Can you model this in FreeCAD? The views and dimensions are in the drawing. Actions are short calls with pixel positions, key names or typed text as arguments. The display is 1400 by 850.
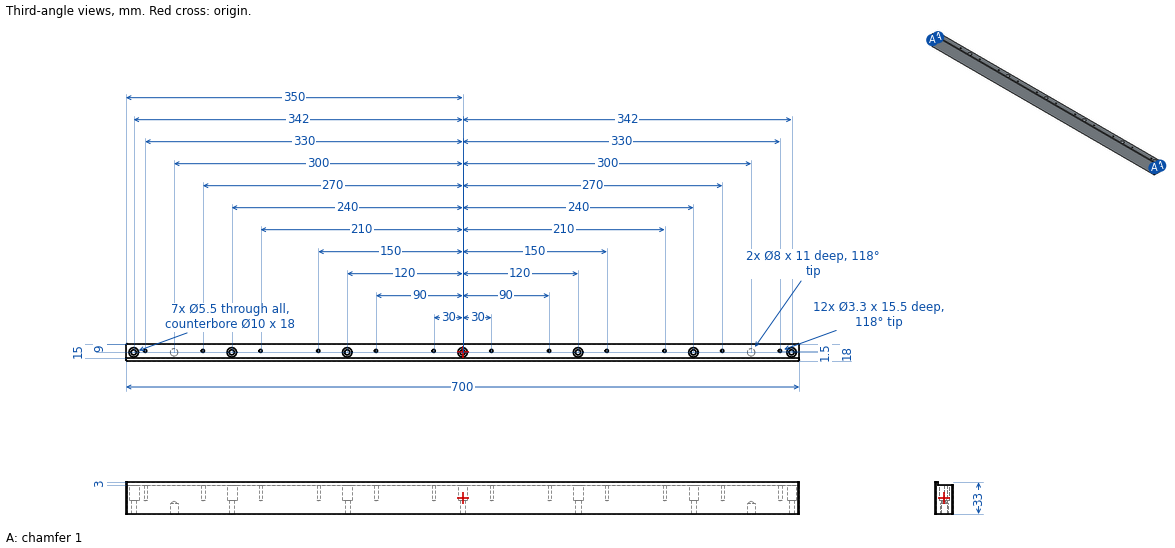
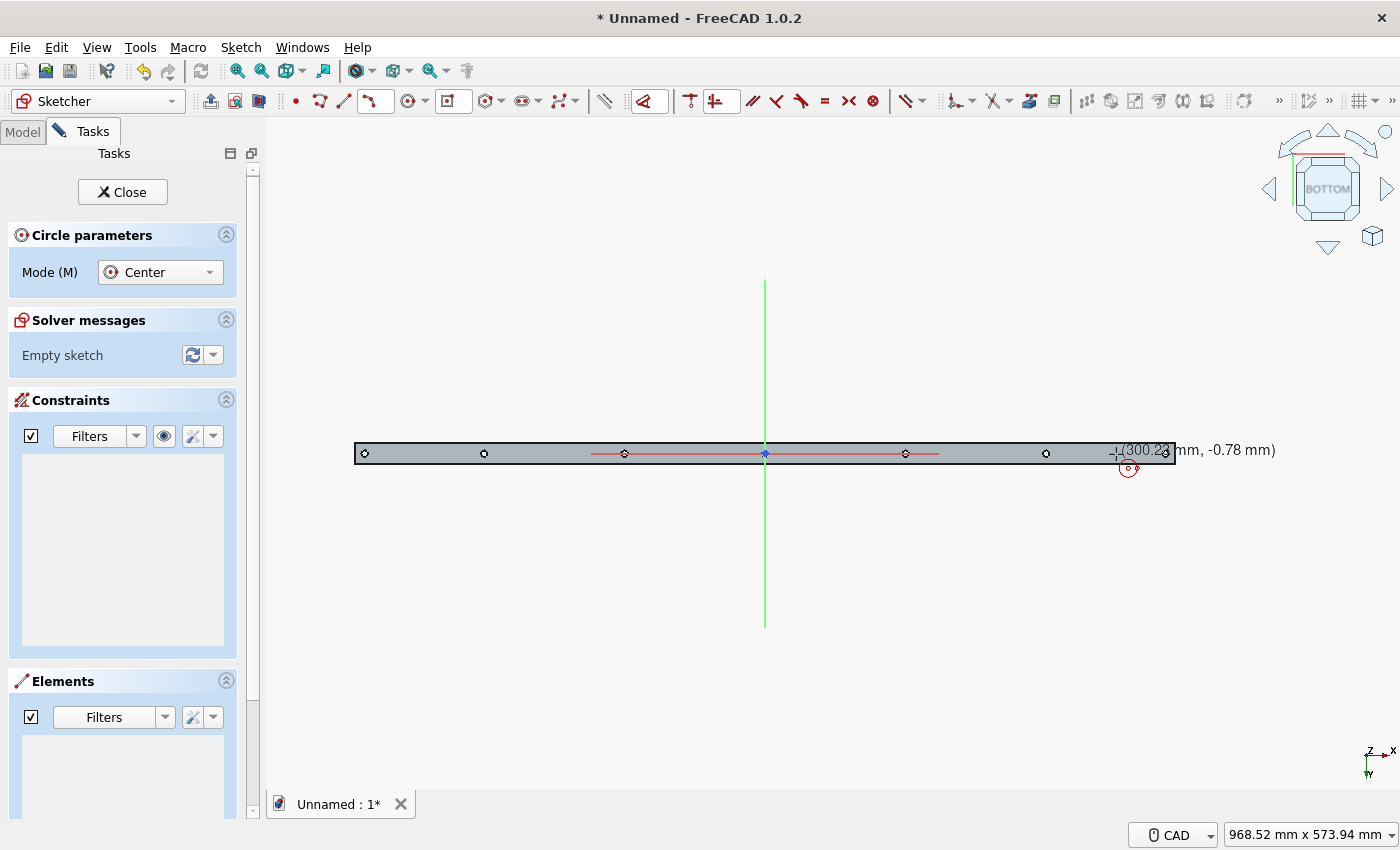
click(1116, 454)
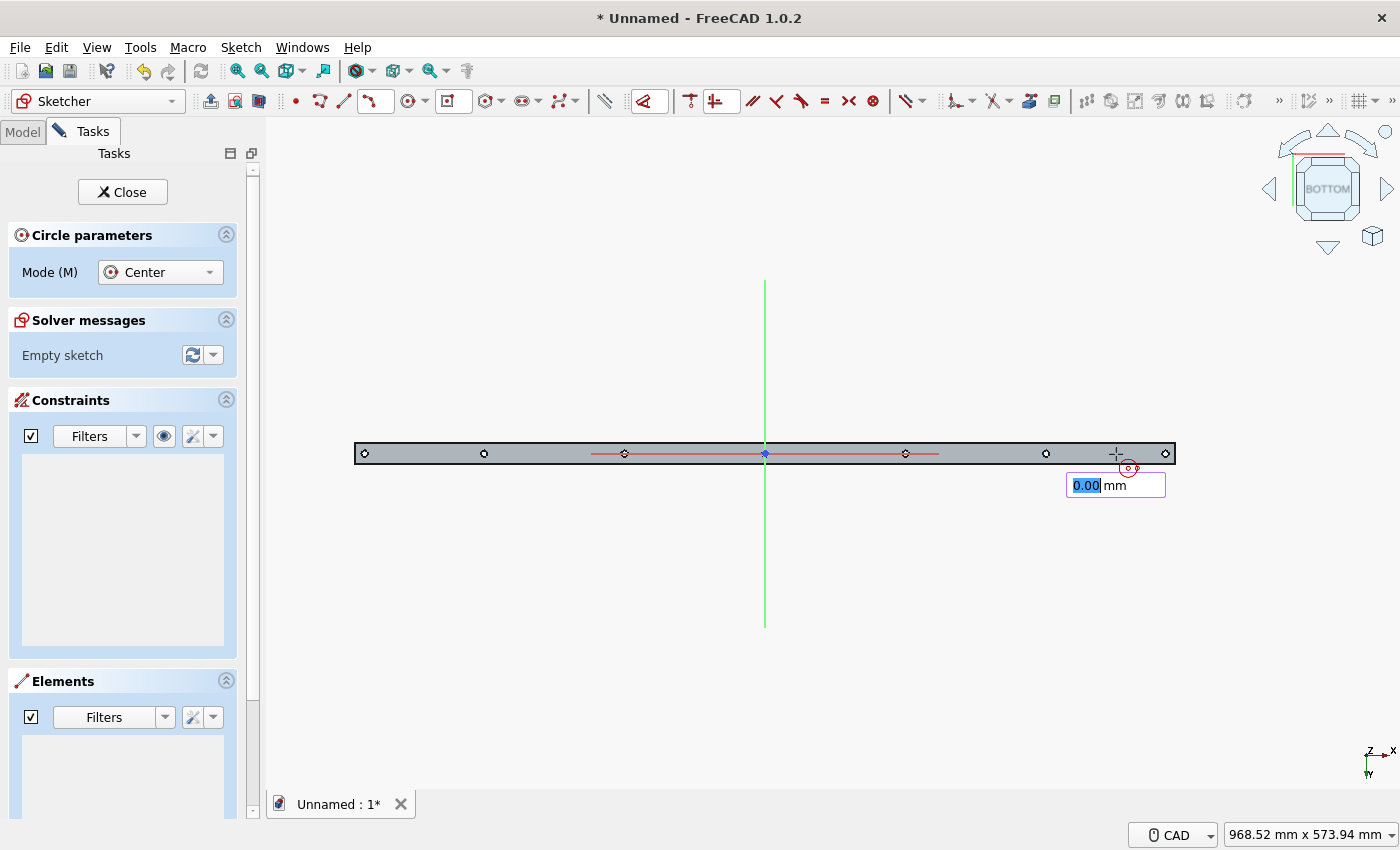
scroll(1115, 458, up, 7)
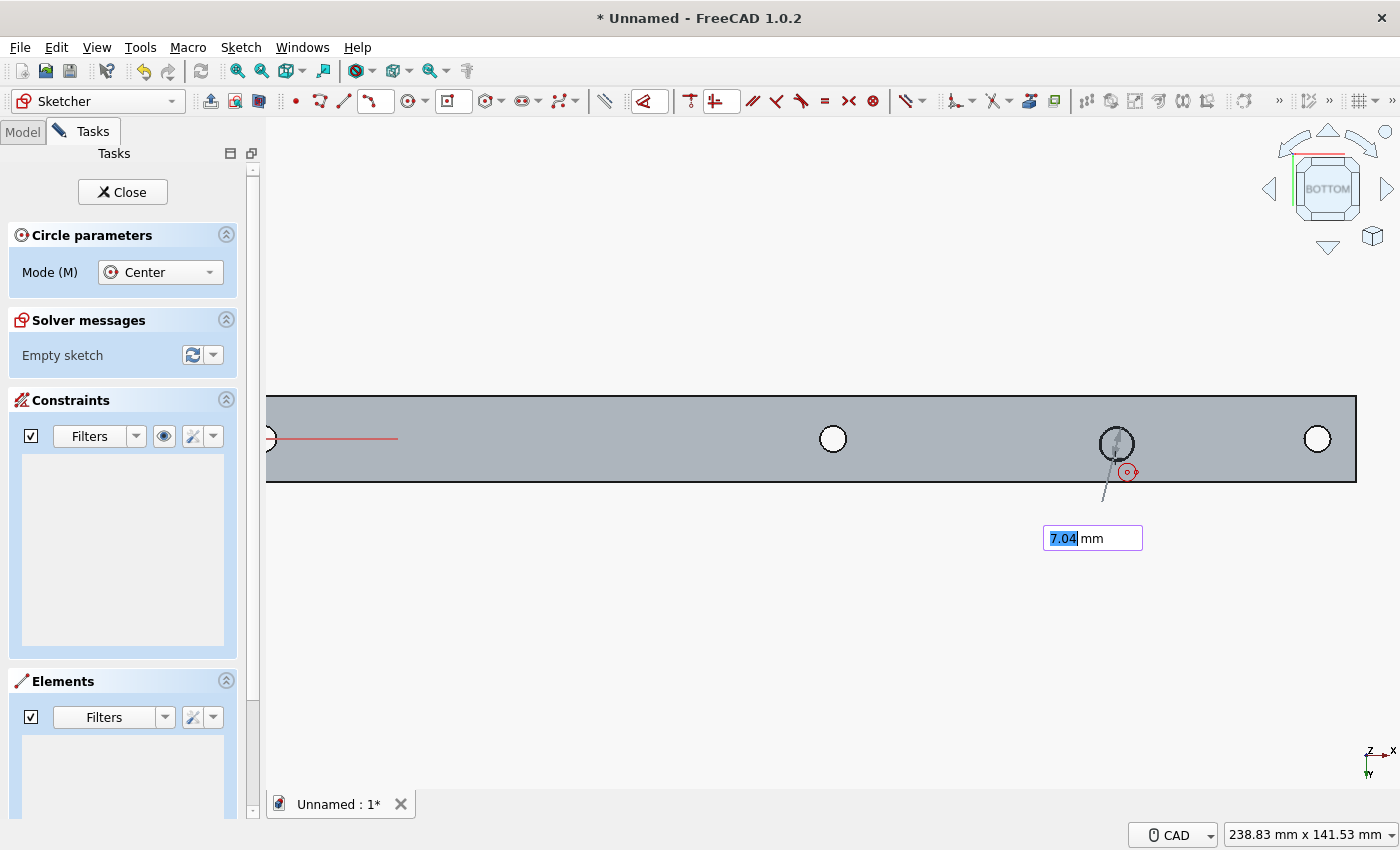
click(1112, 457)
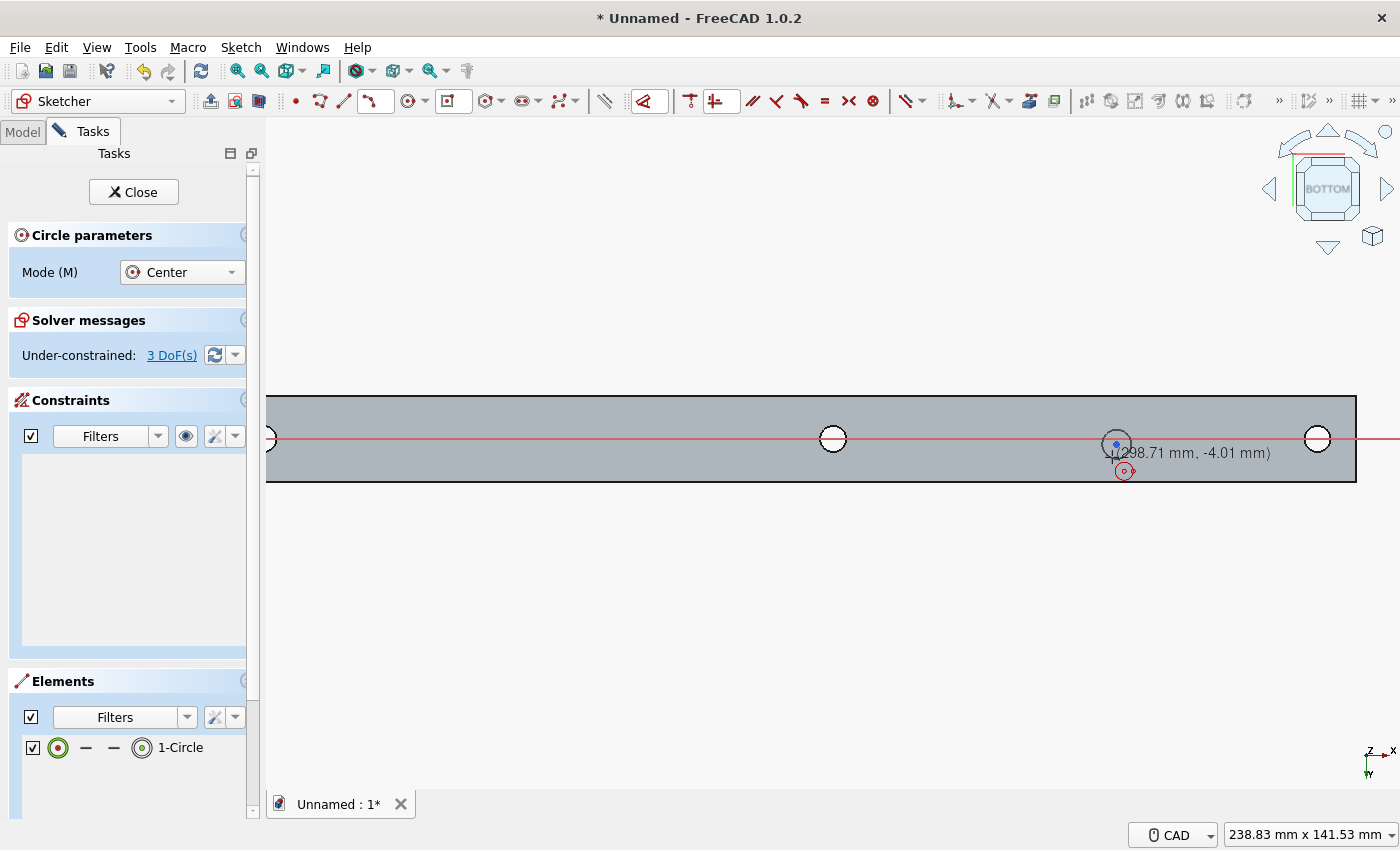
scroll(1115, 458, down, 7)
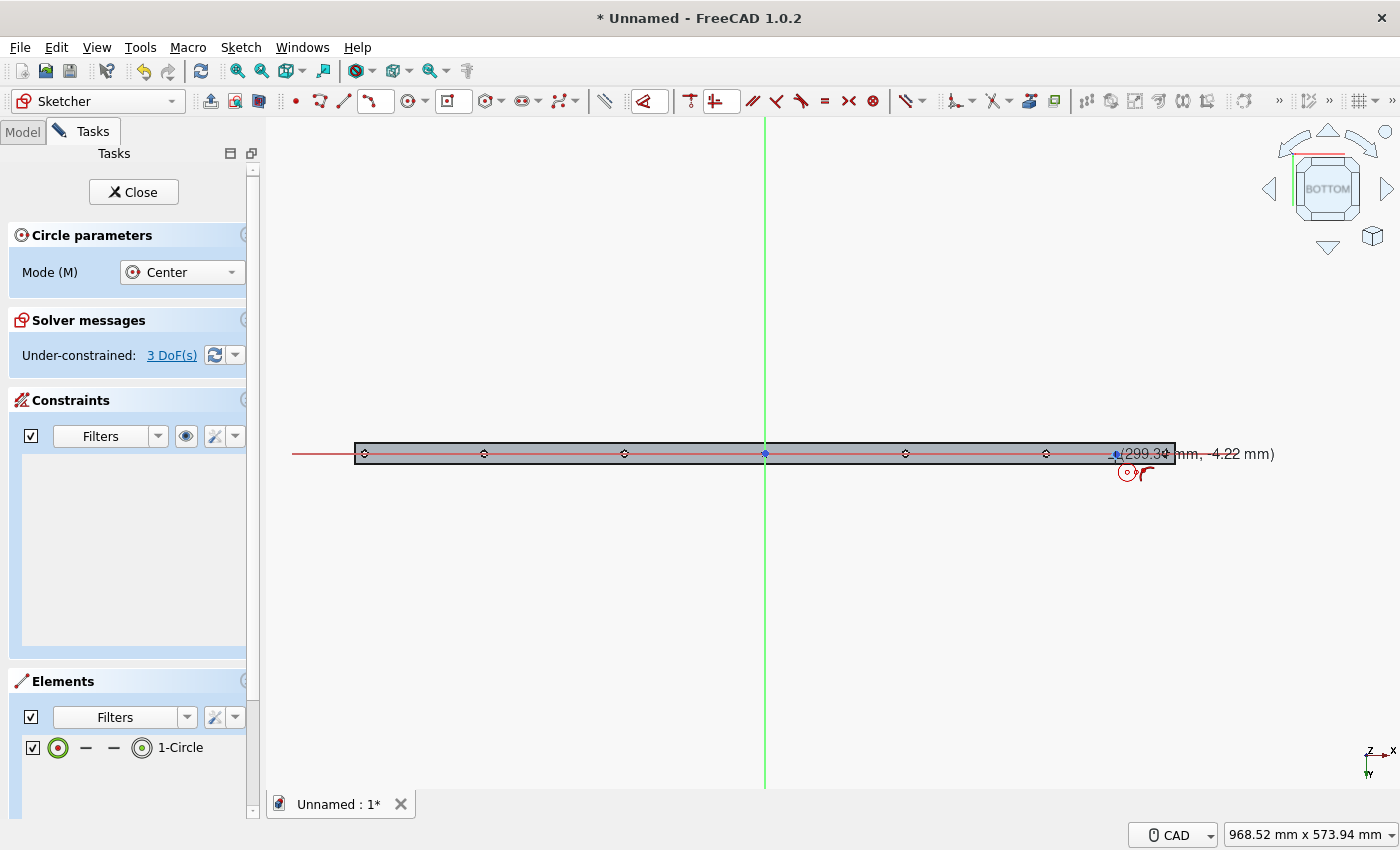
scroll(414, 454, up, 8)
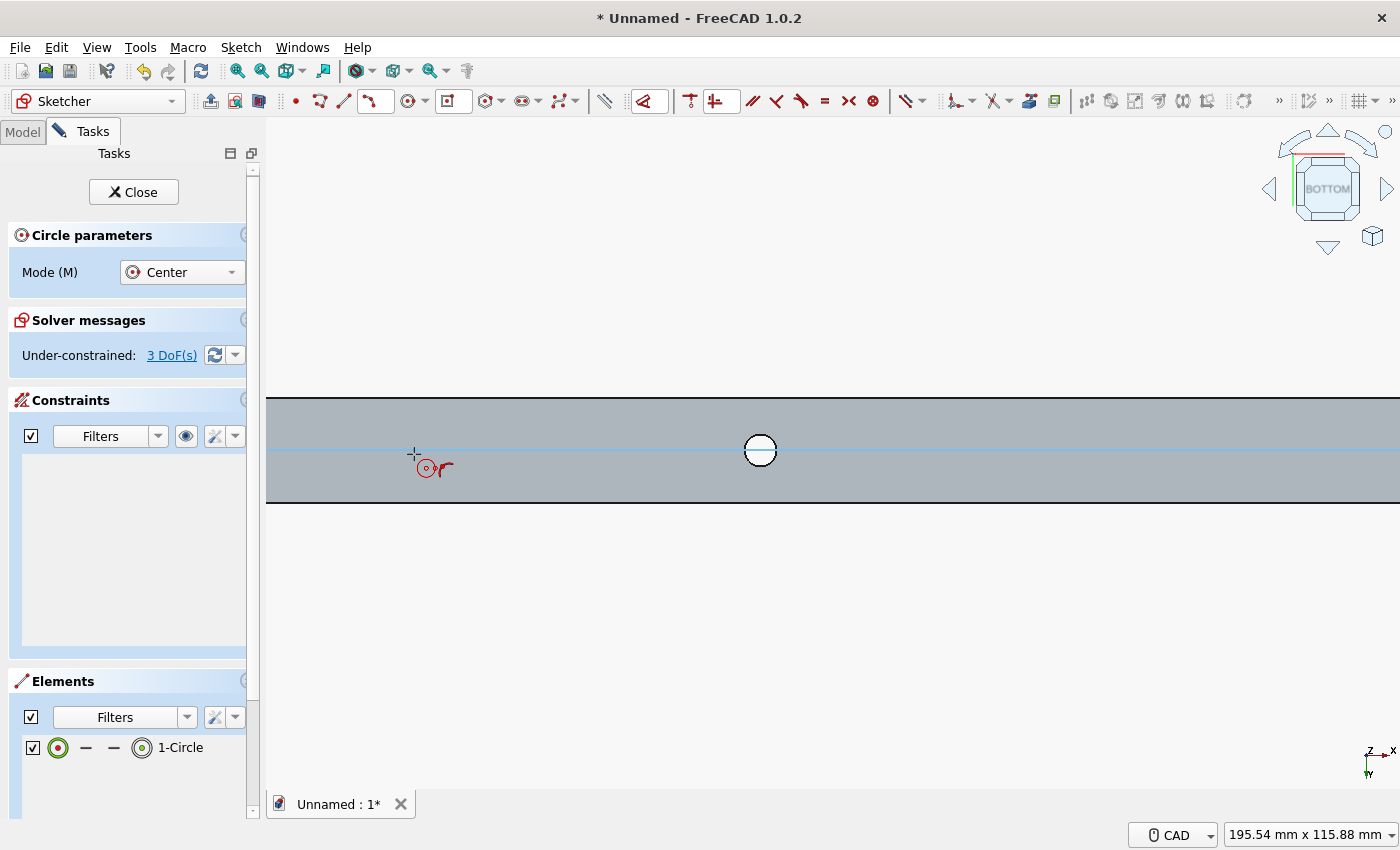
scroll(413, 454, down, 8)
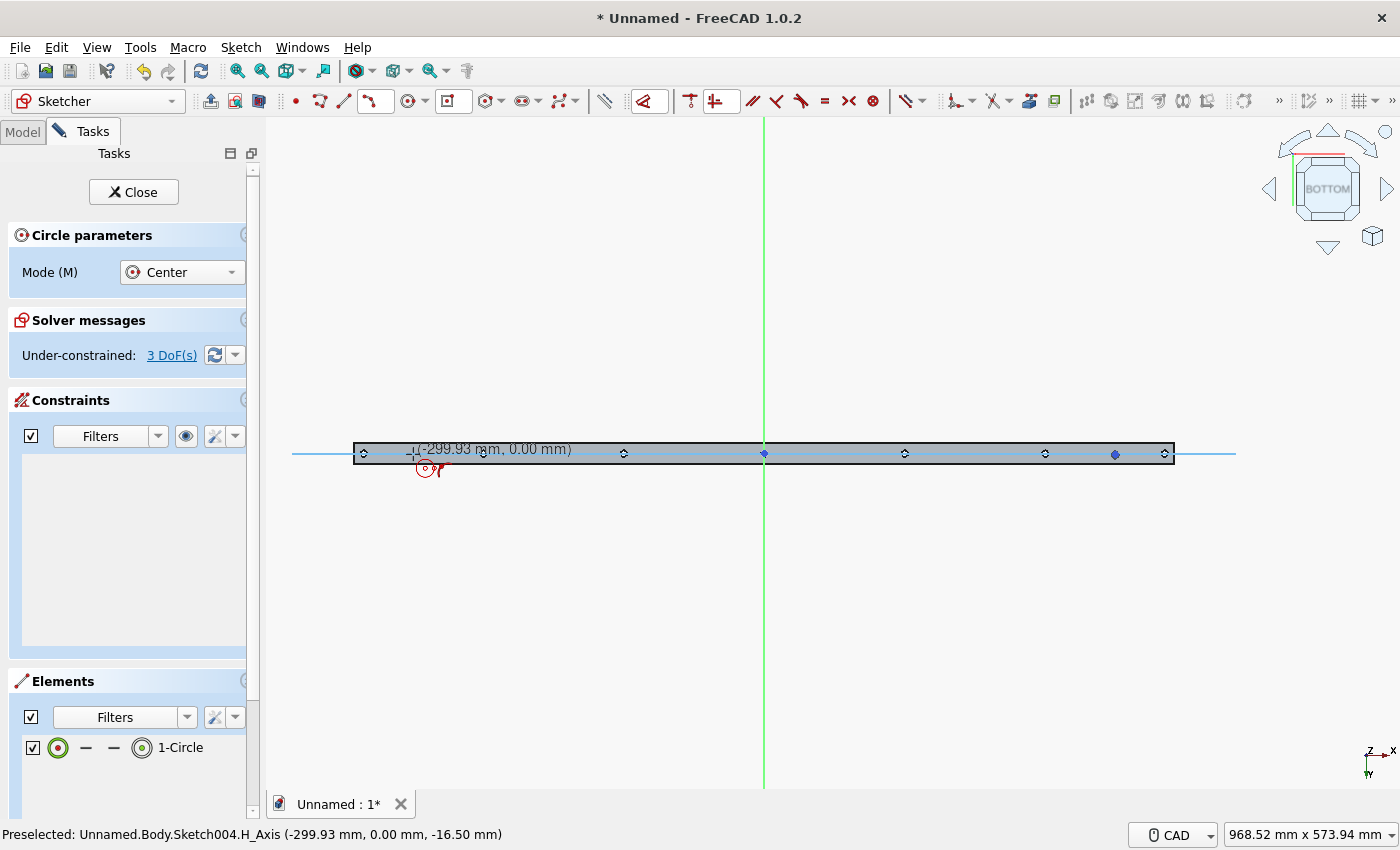
click(413, 454)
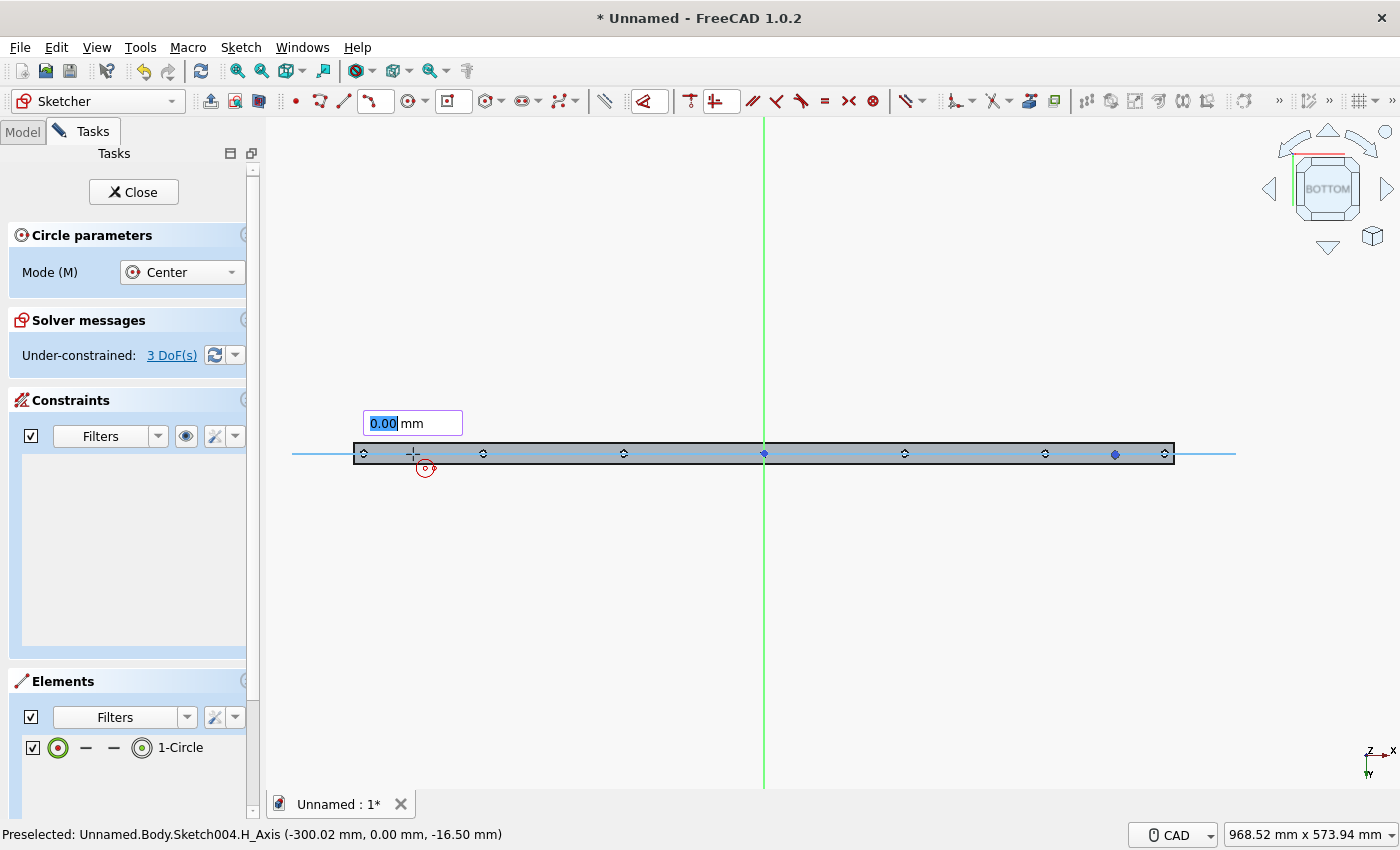
scroll(411, 458, up, 7)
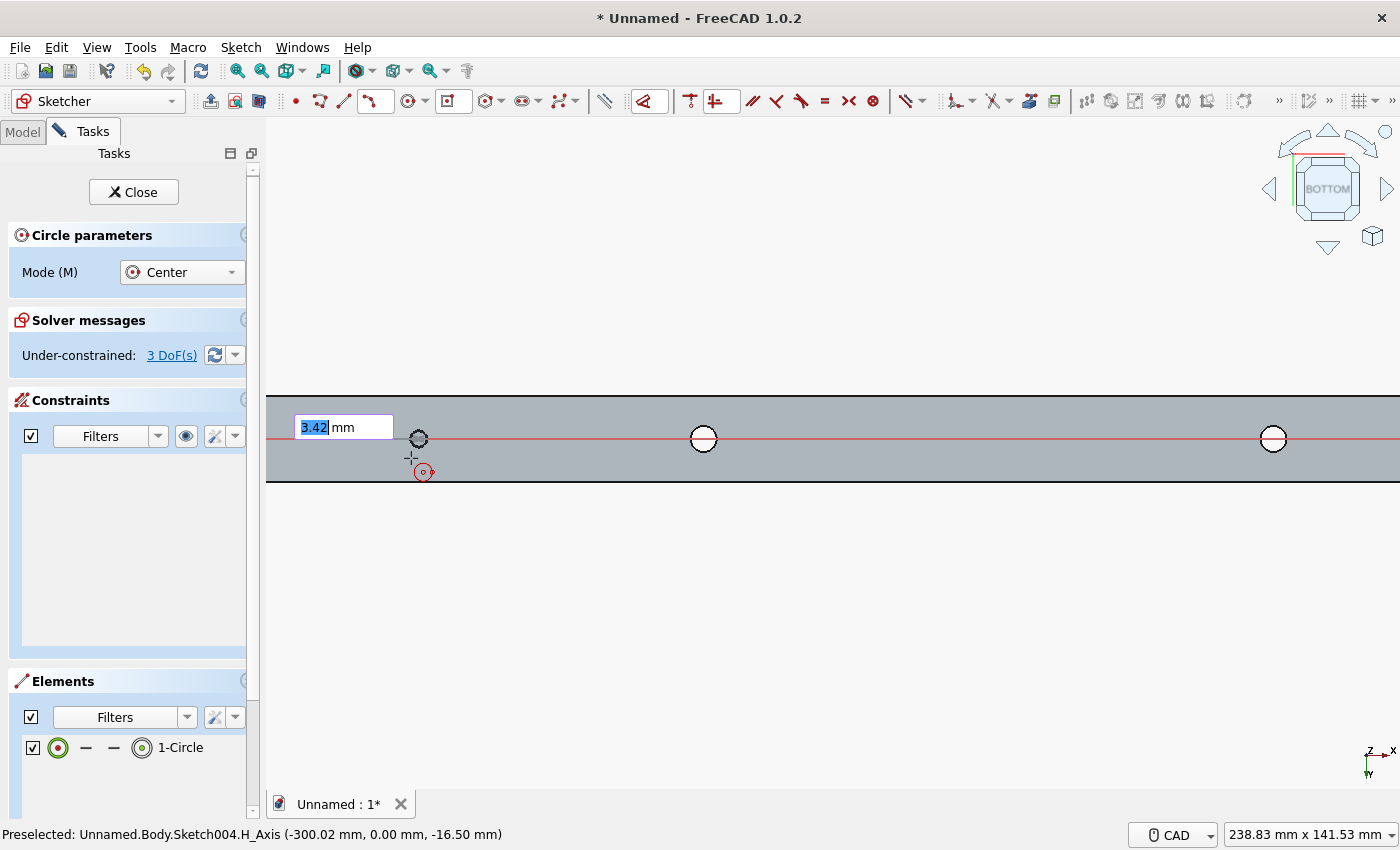
click(412, 457)
key(Escape)